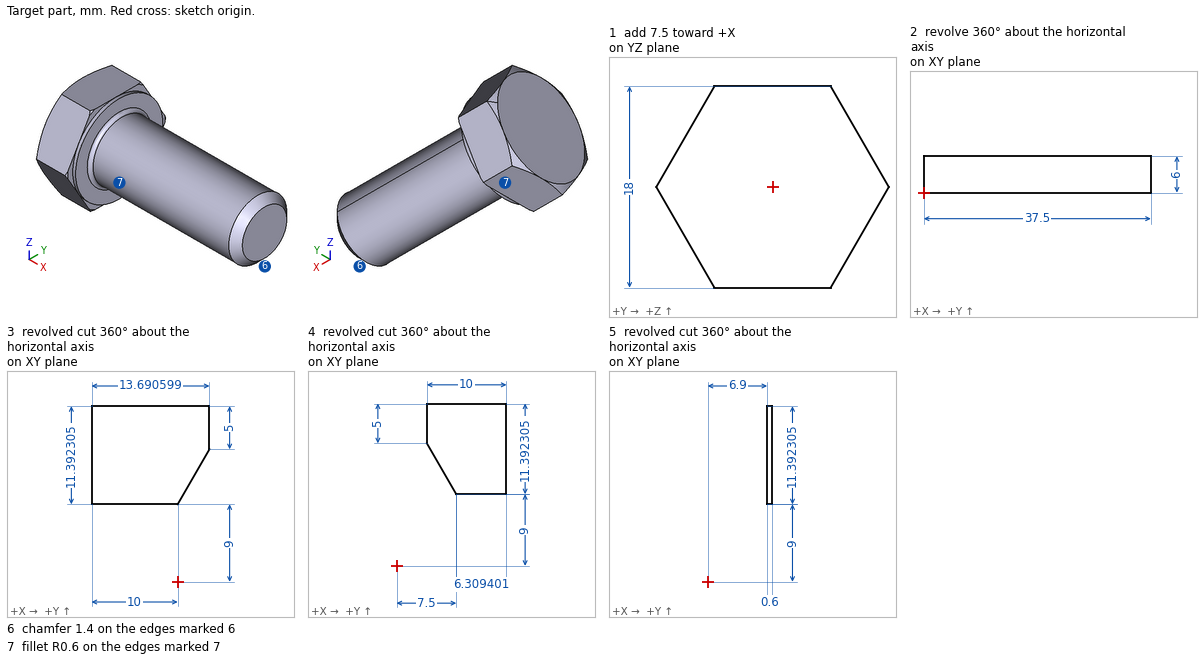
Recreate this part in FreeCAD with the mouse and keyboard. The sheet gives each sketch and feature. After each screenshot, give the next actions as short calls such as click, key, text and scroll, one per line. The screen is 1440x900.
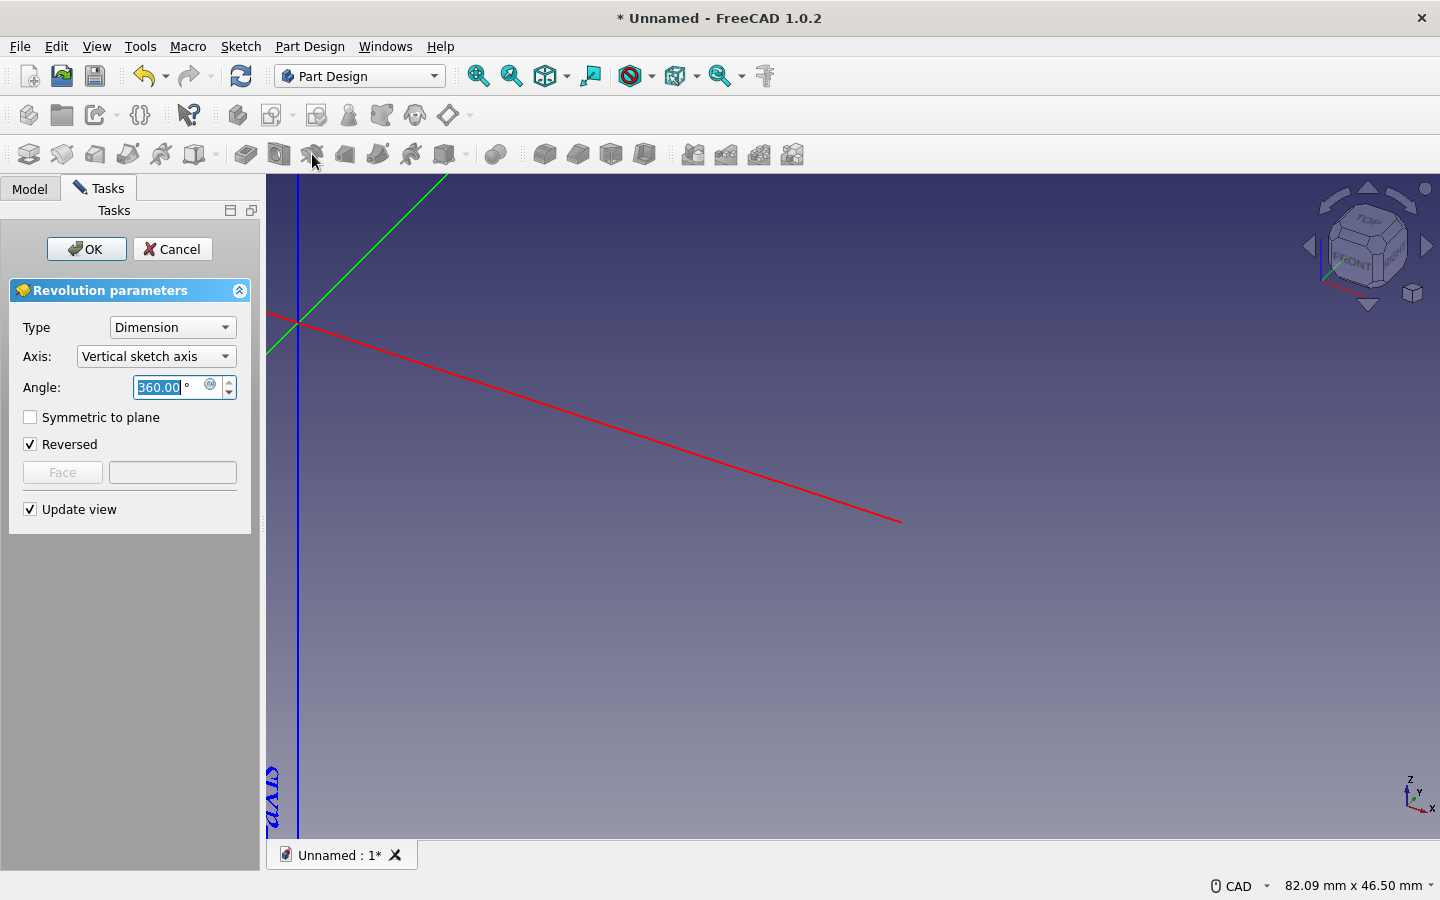
click(157, 356)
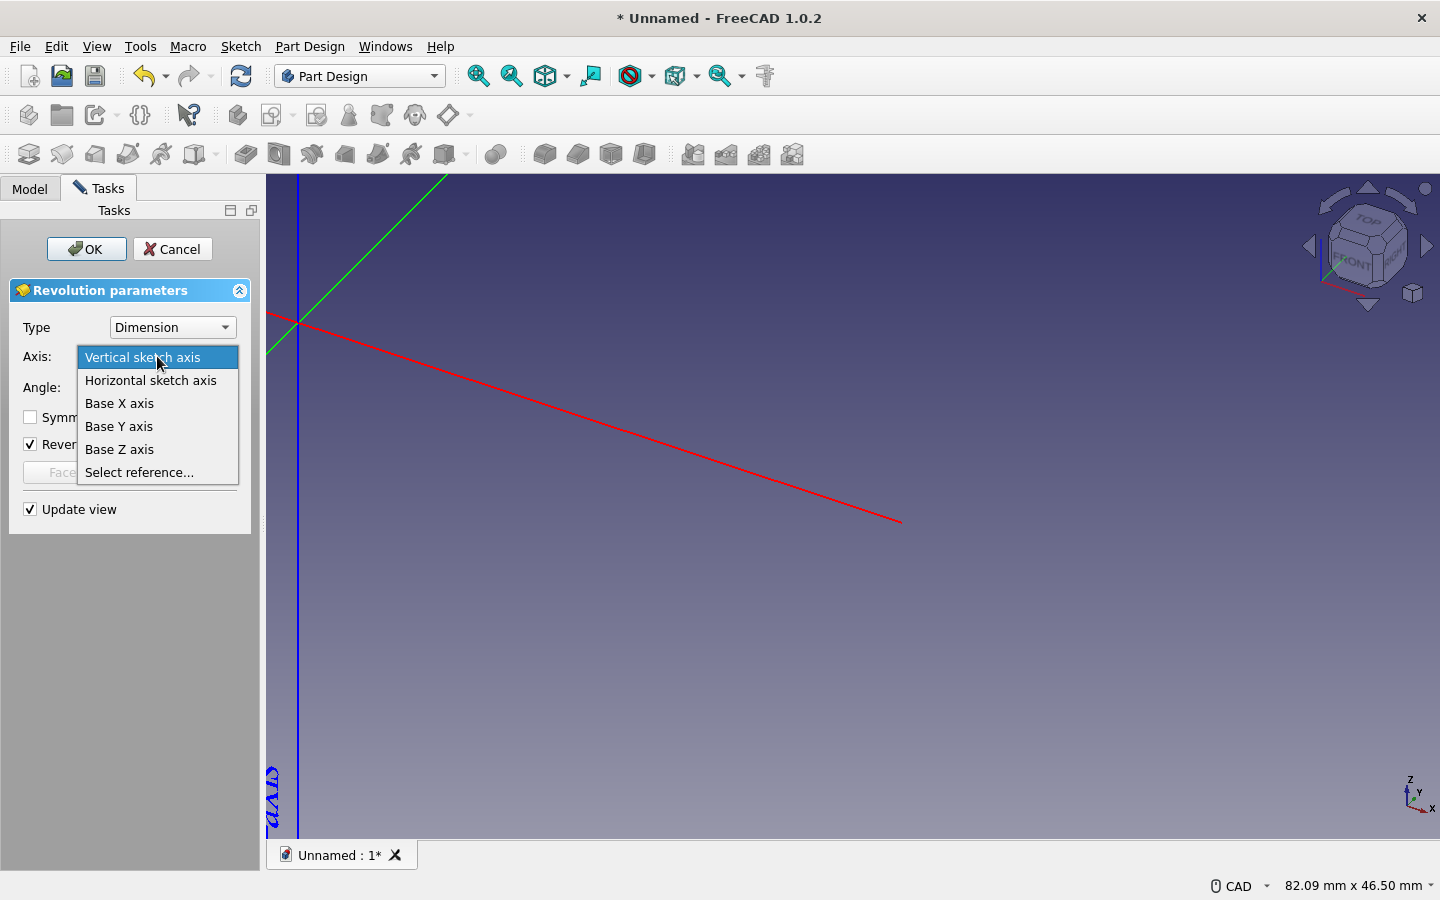
click(156, 380)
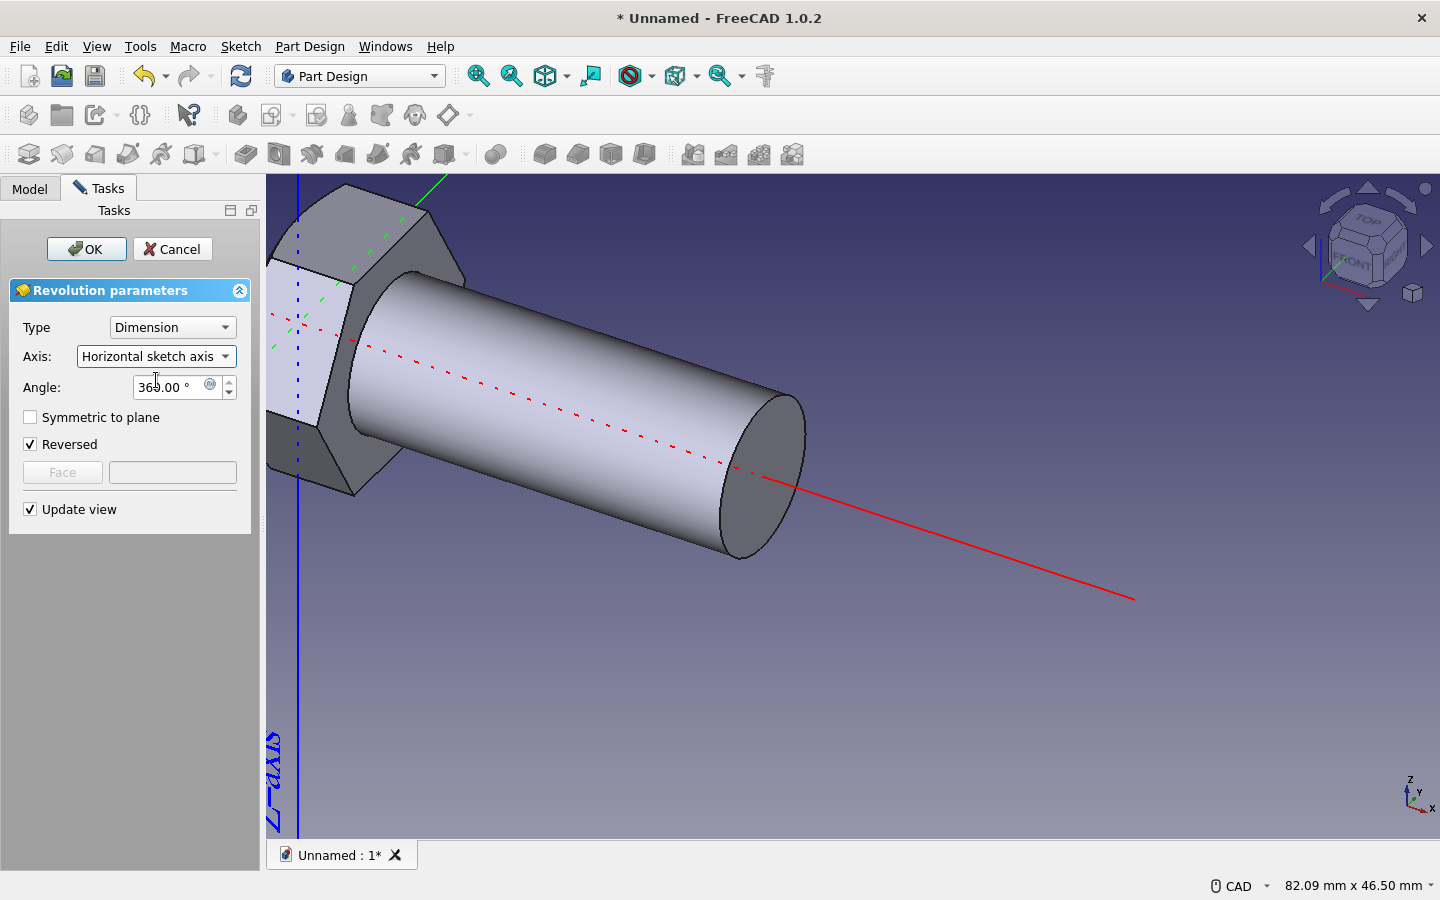
click(87, 249)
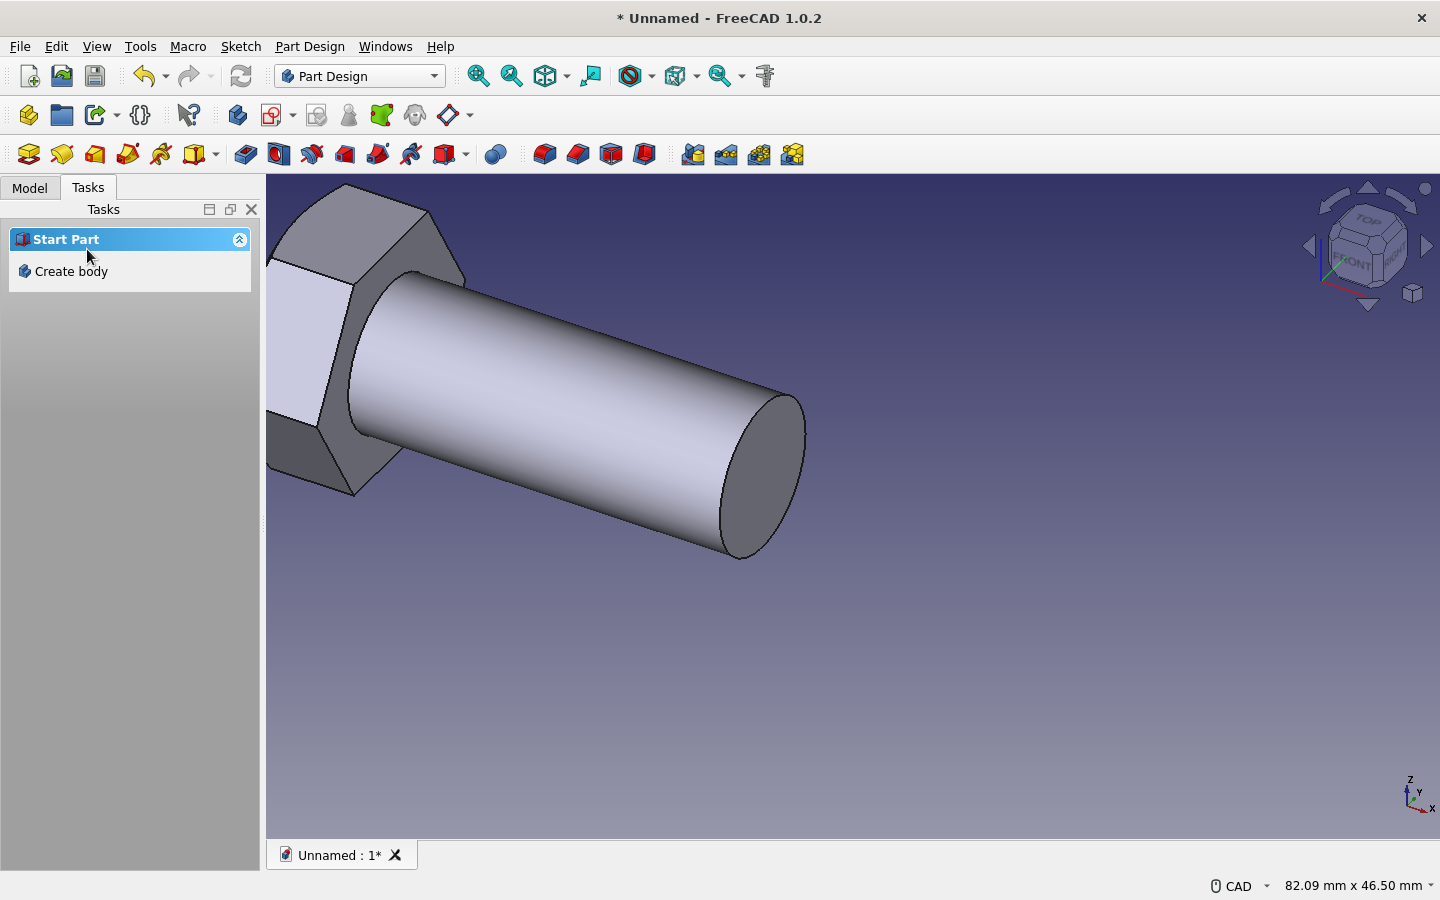
key(v)
key(f)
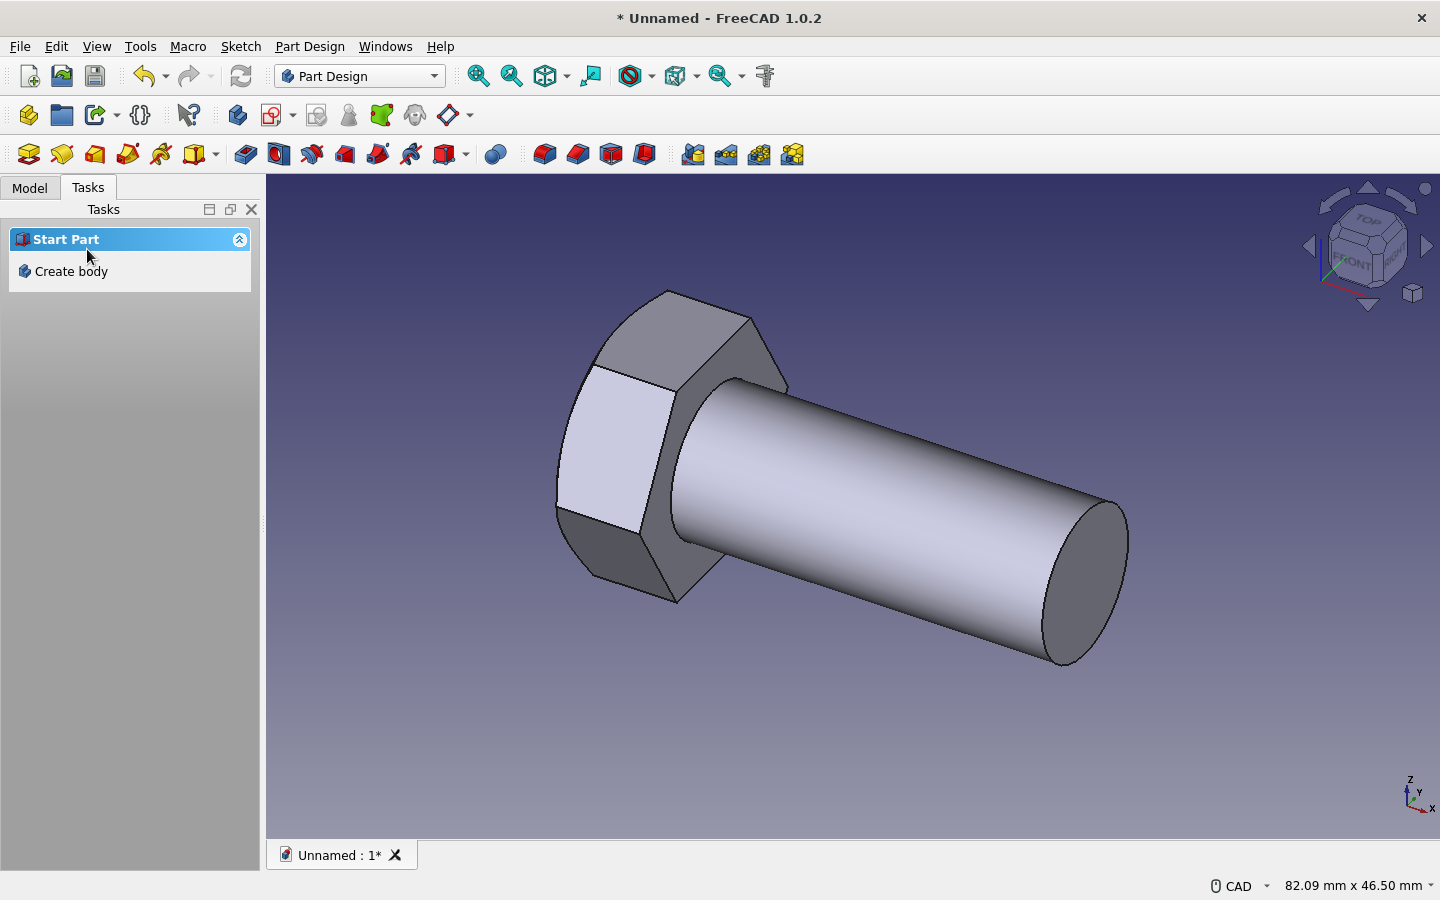
click(270, 116)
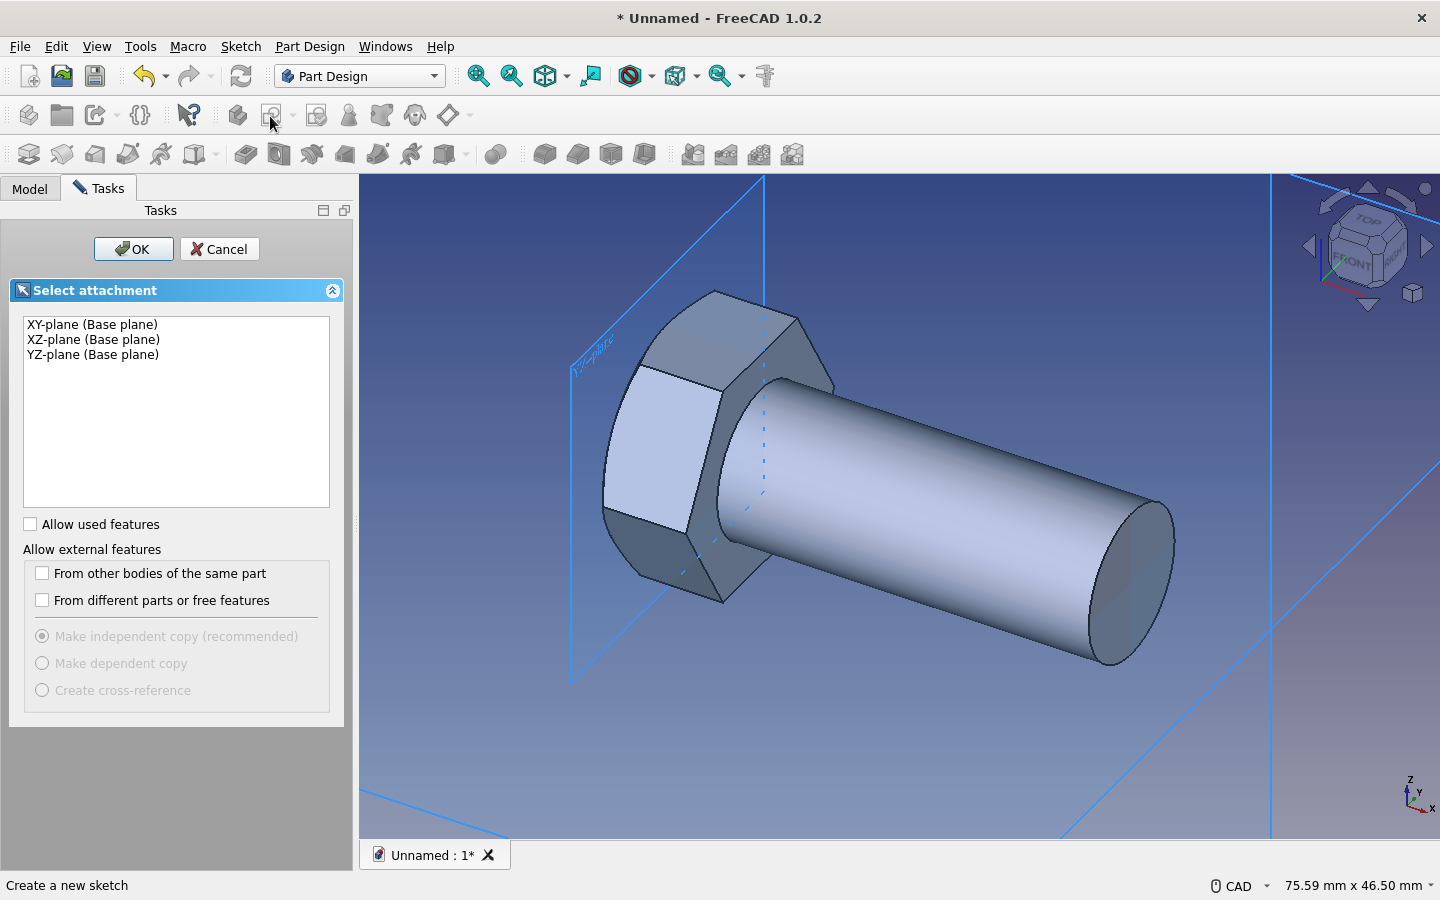
click(84, 324)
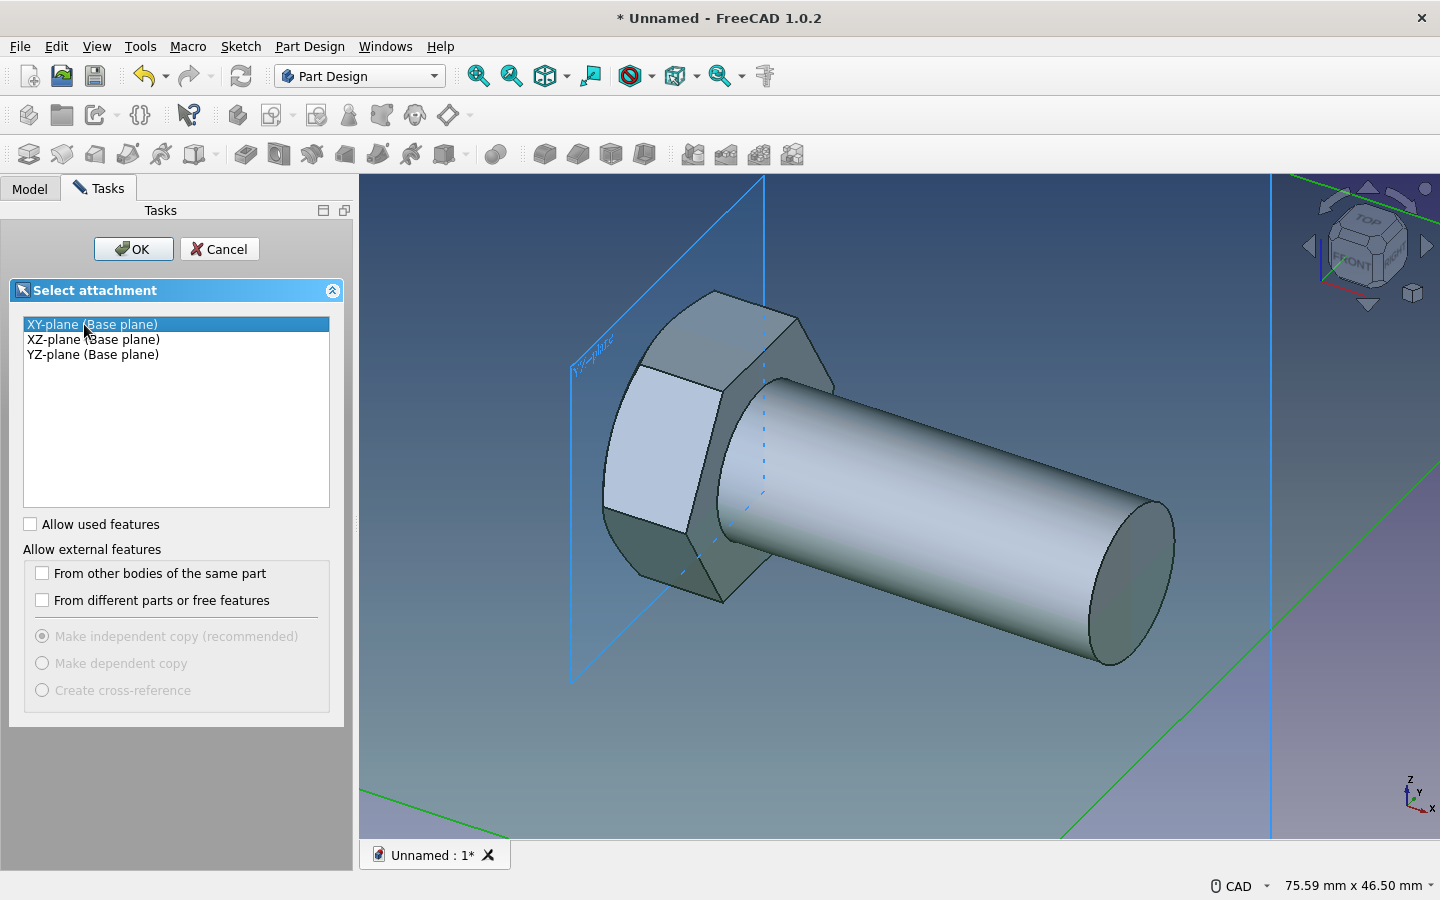
click(134, 249)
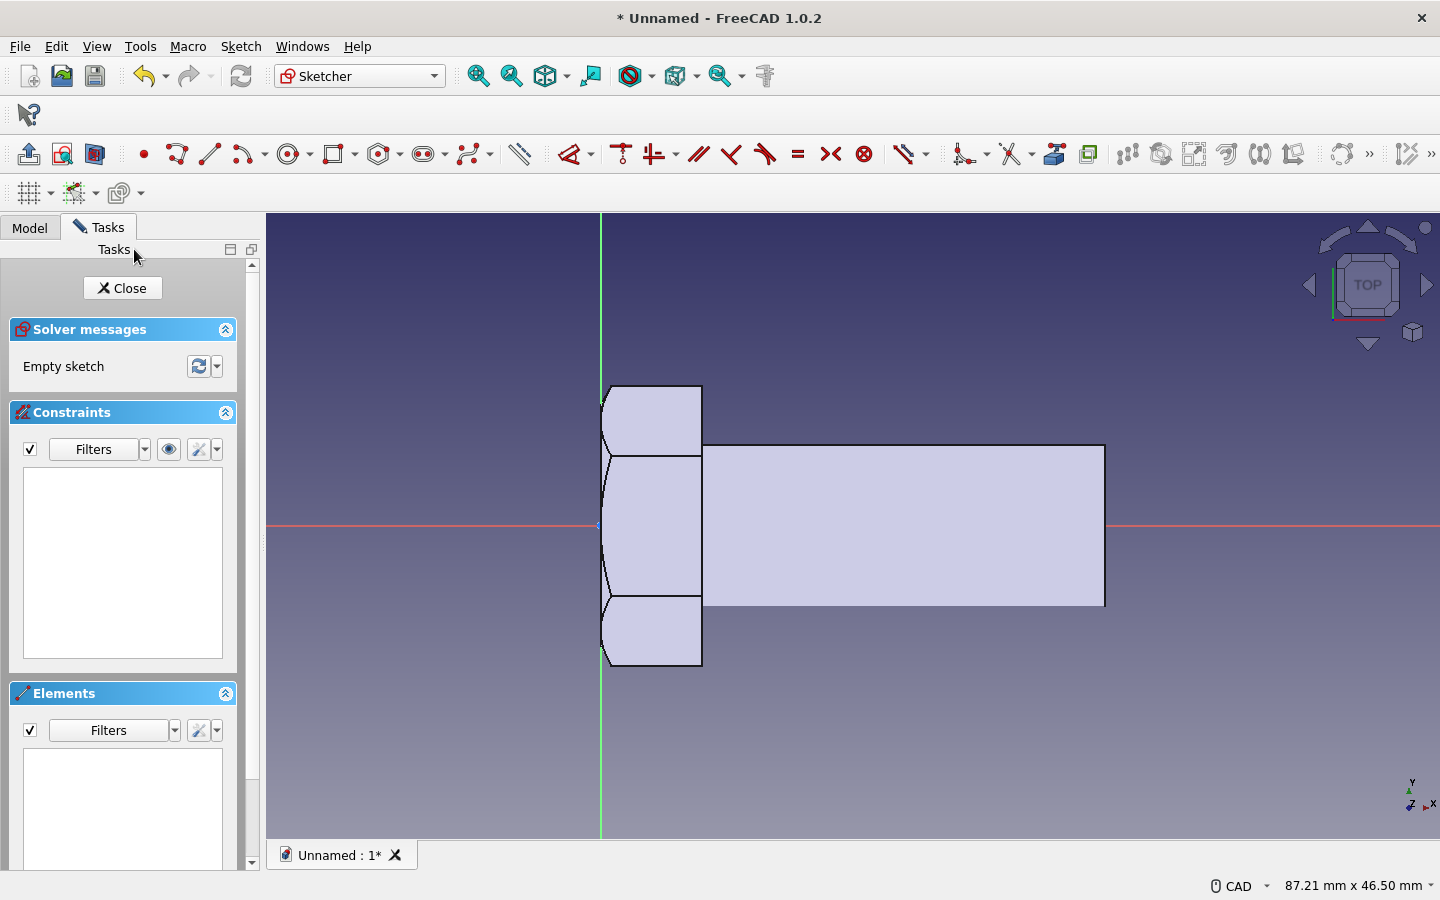
key(q)
key(s)